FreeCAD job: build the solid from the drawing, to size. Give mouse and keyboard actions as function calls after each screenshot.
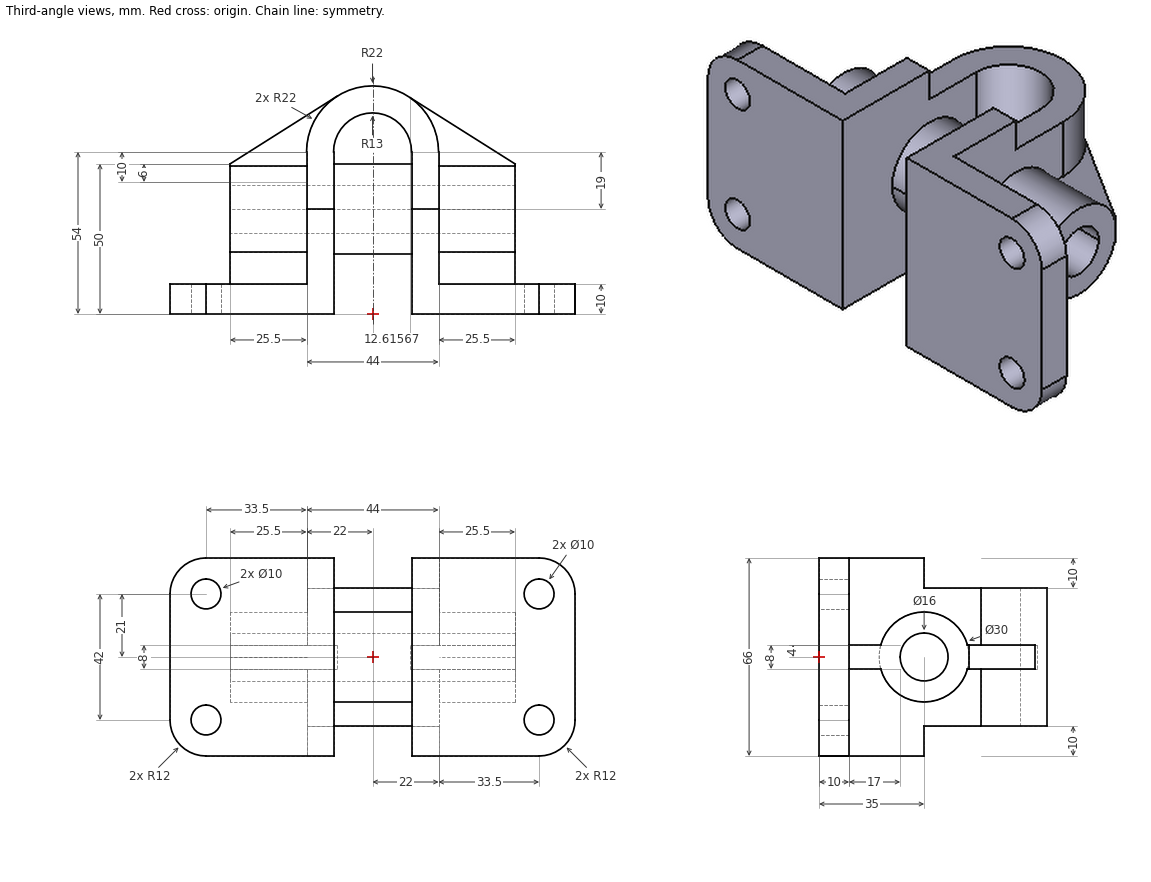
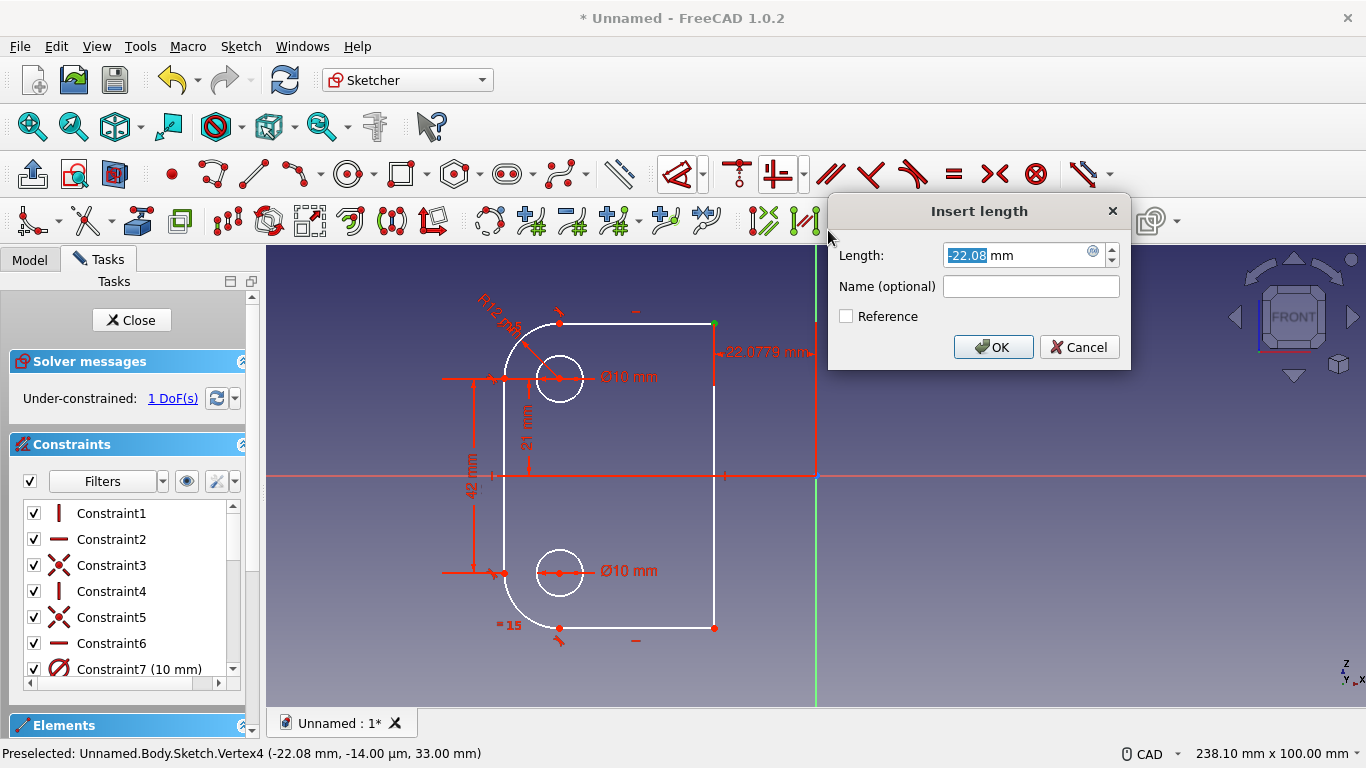
text(-22)
key(Return)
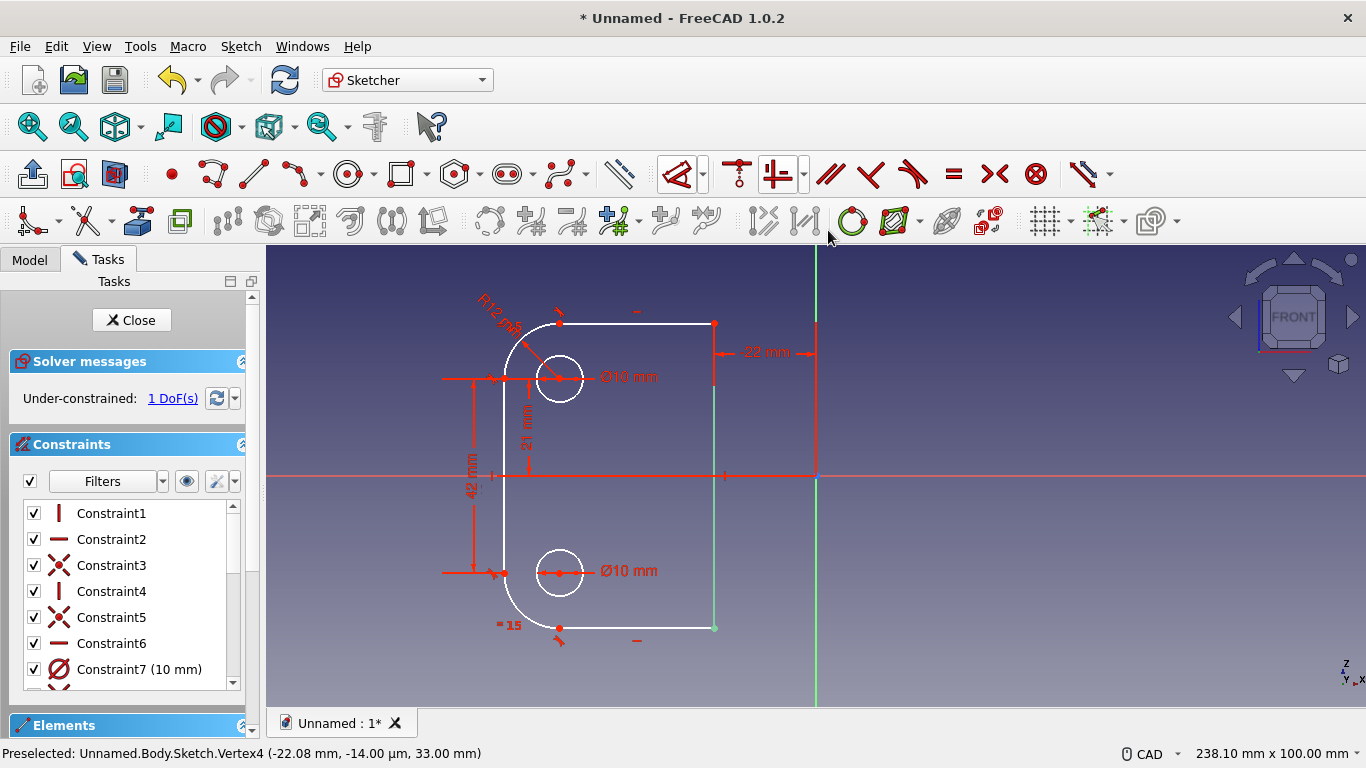
click(606, 324)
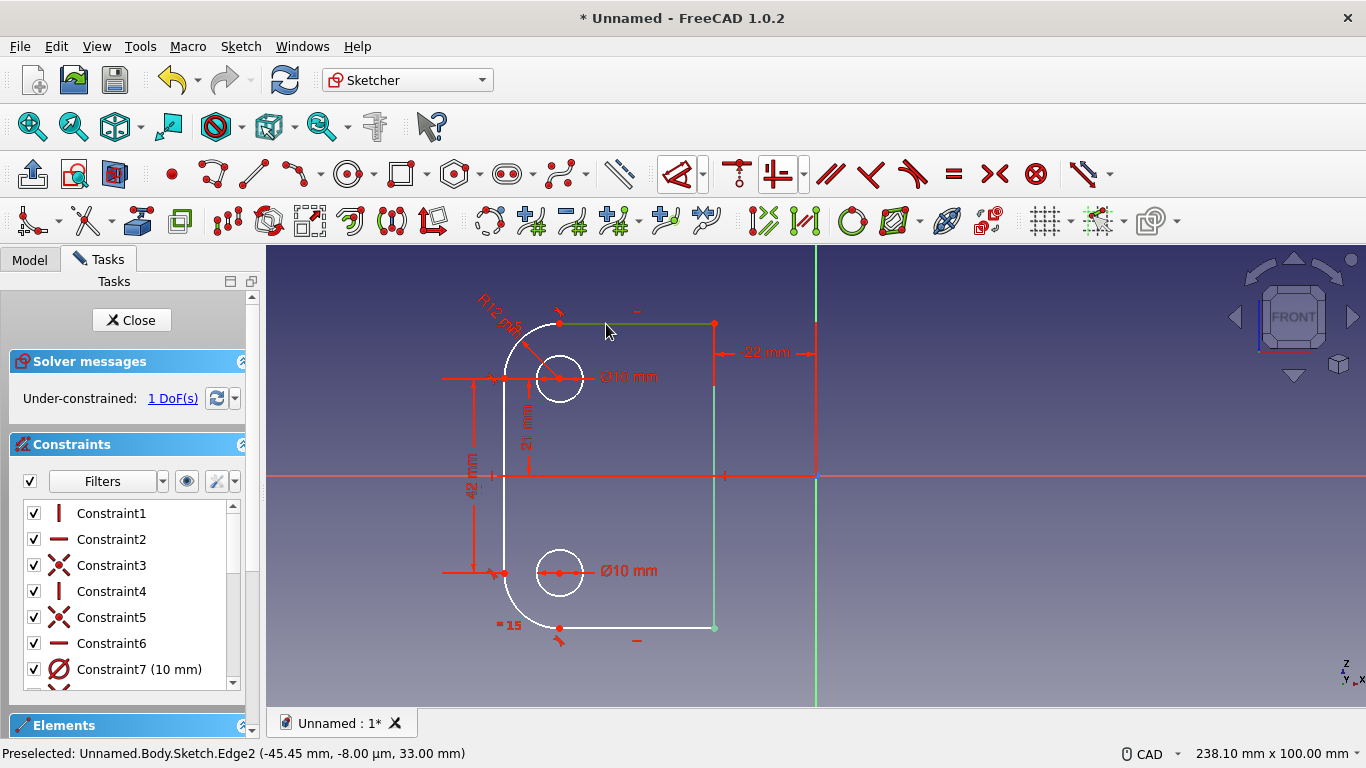
click(702, 174)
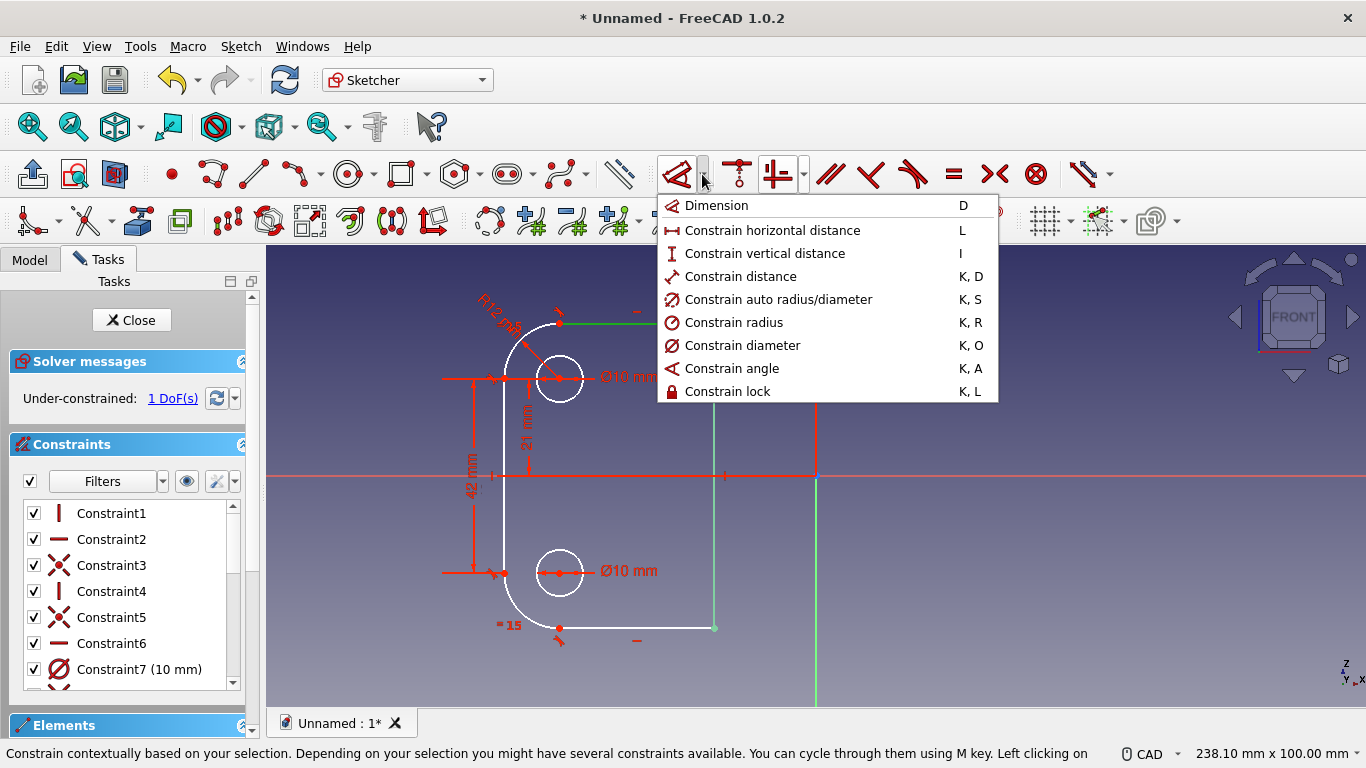
click(828, 230)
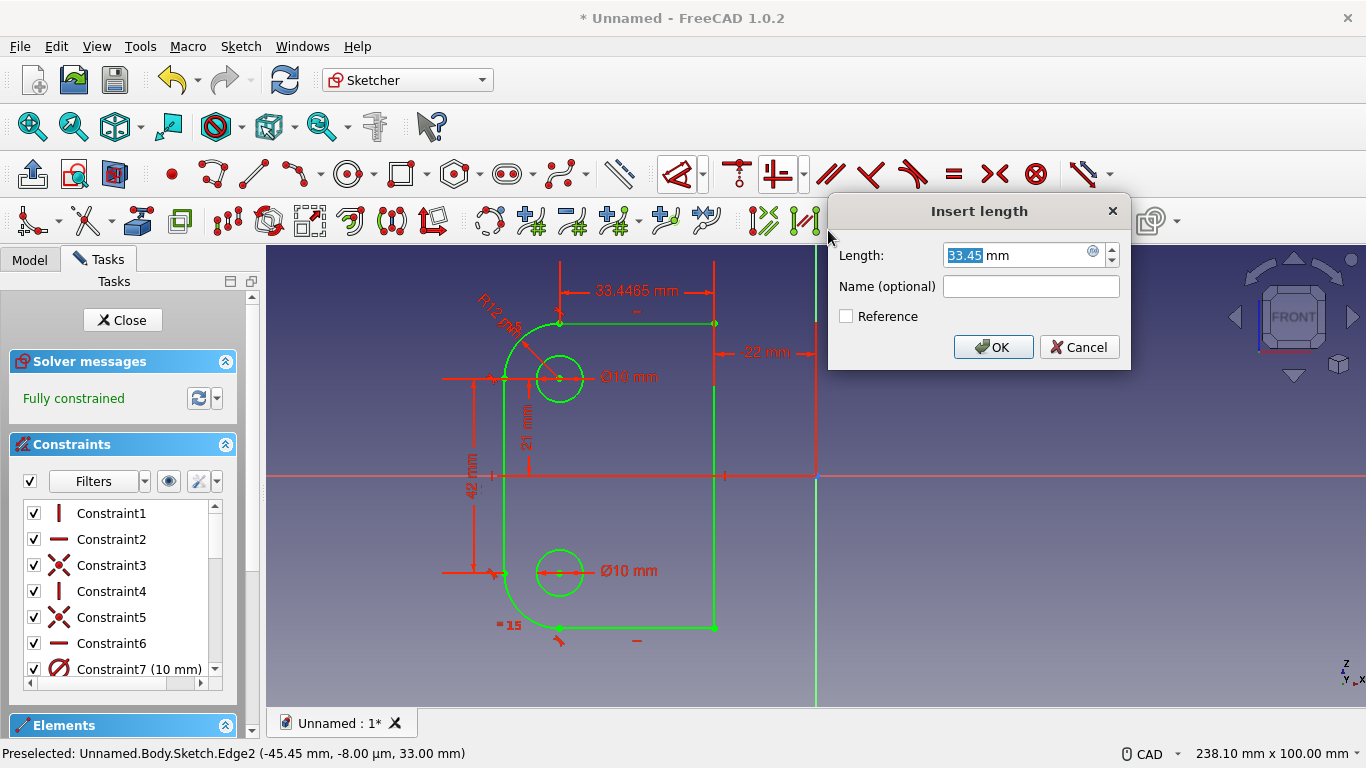
text(33.5)
key(Return)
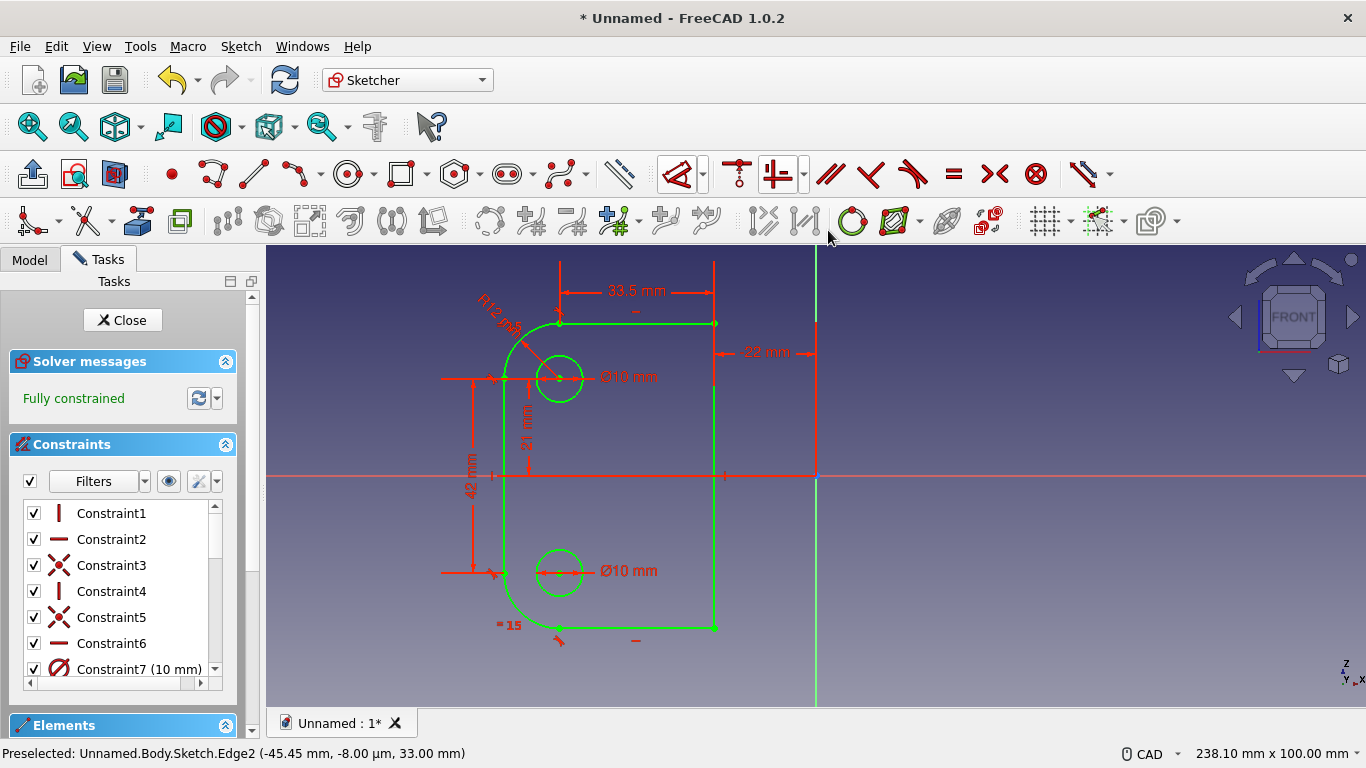
click(123, 320)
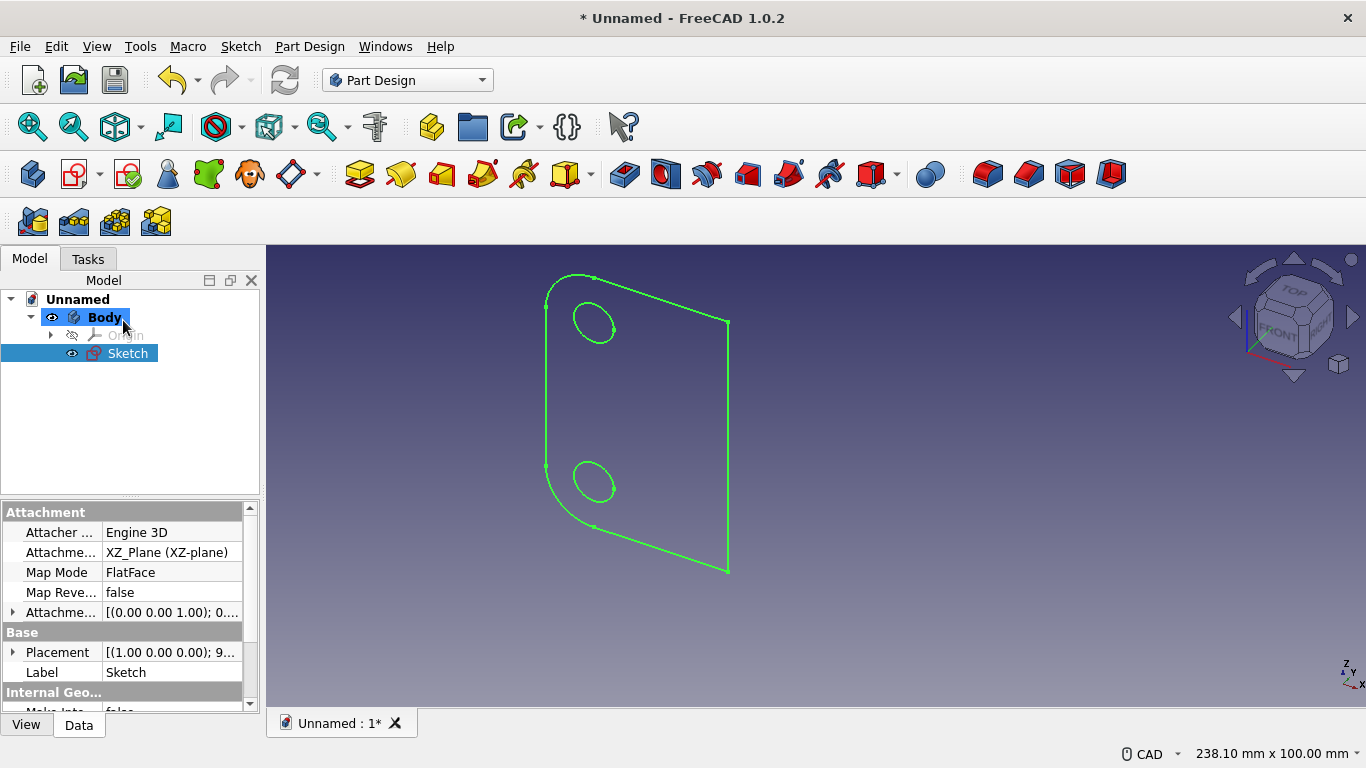
click(360, 174)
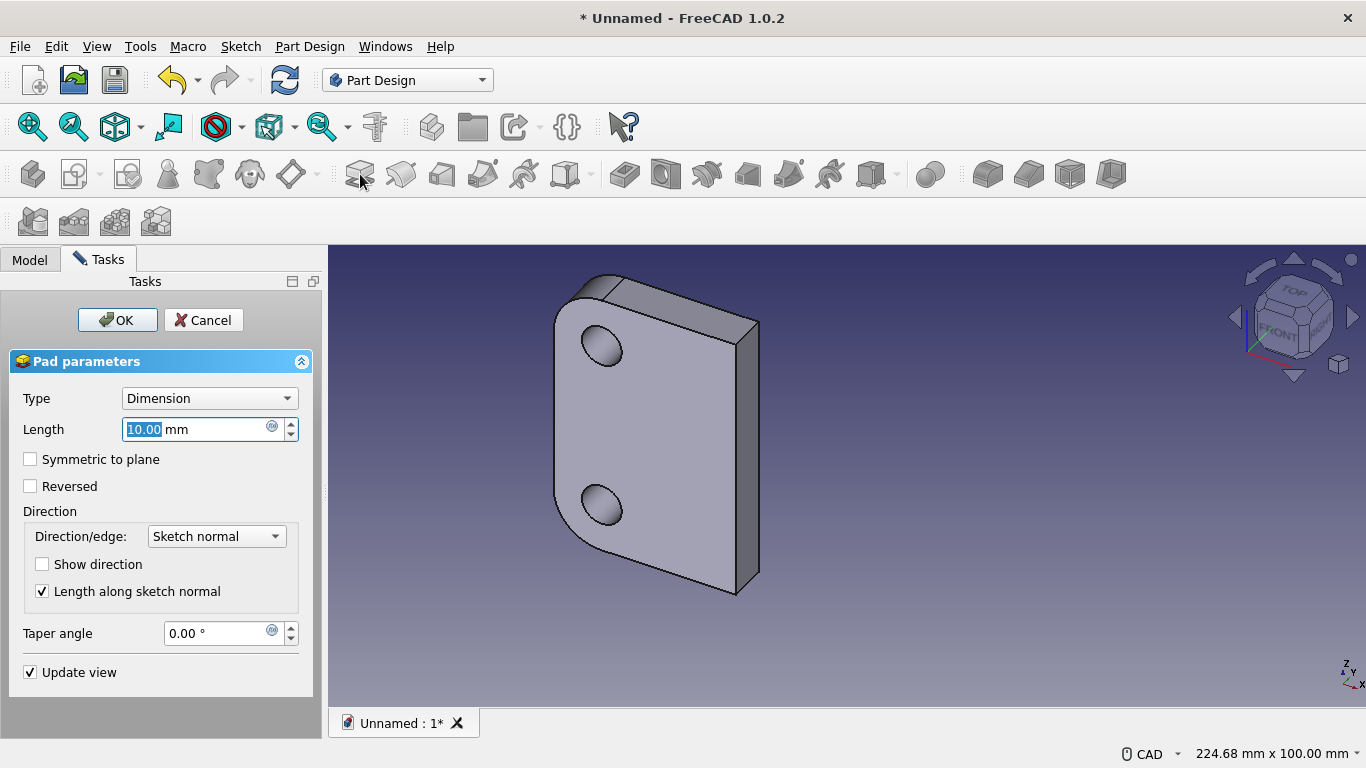
text(10)
key(Tab)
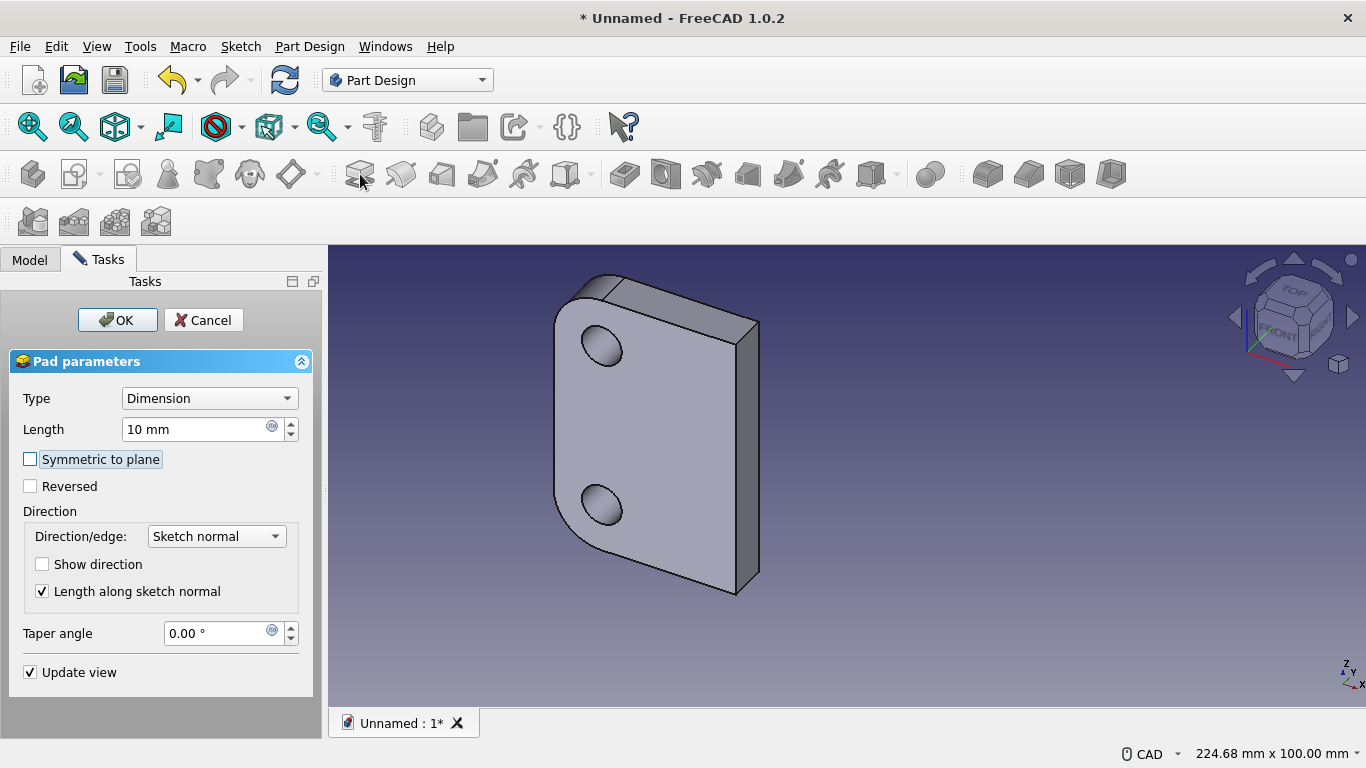
click(31, 486)